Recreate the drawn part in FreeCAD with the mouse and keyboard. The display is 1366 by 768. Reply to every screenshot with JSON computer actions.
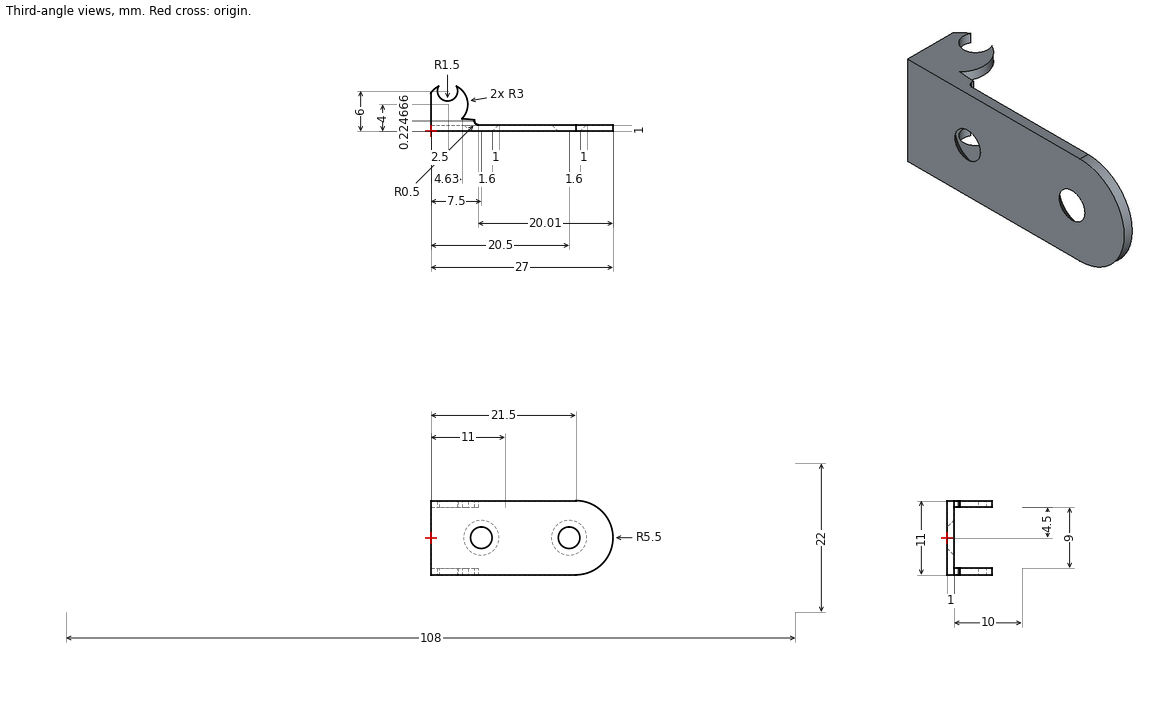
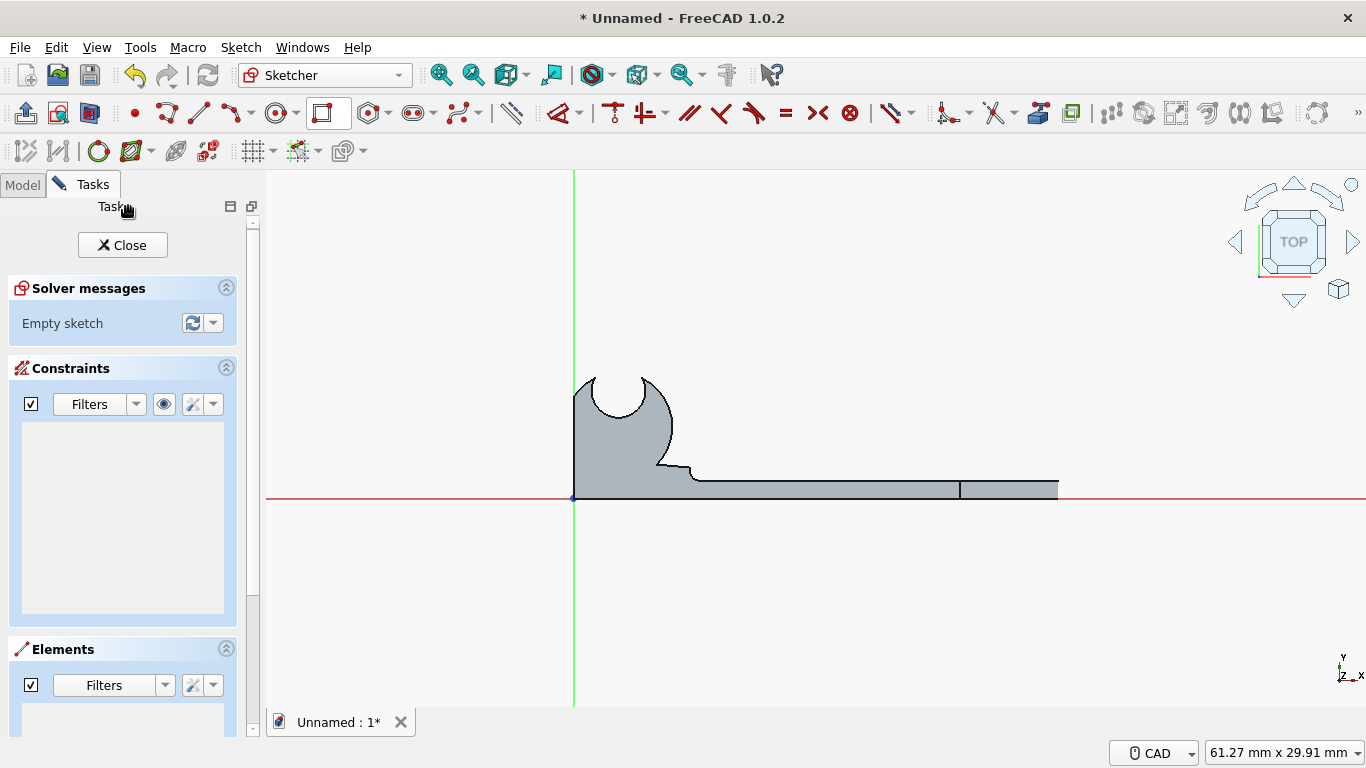
{"action": "key", "text": "q s"}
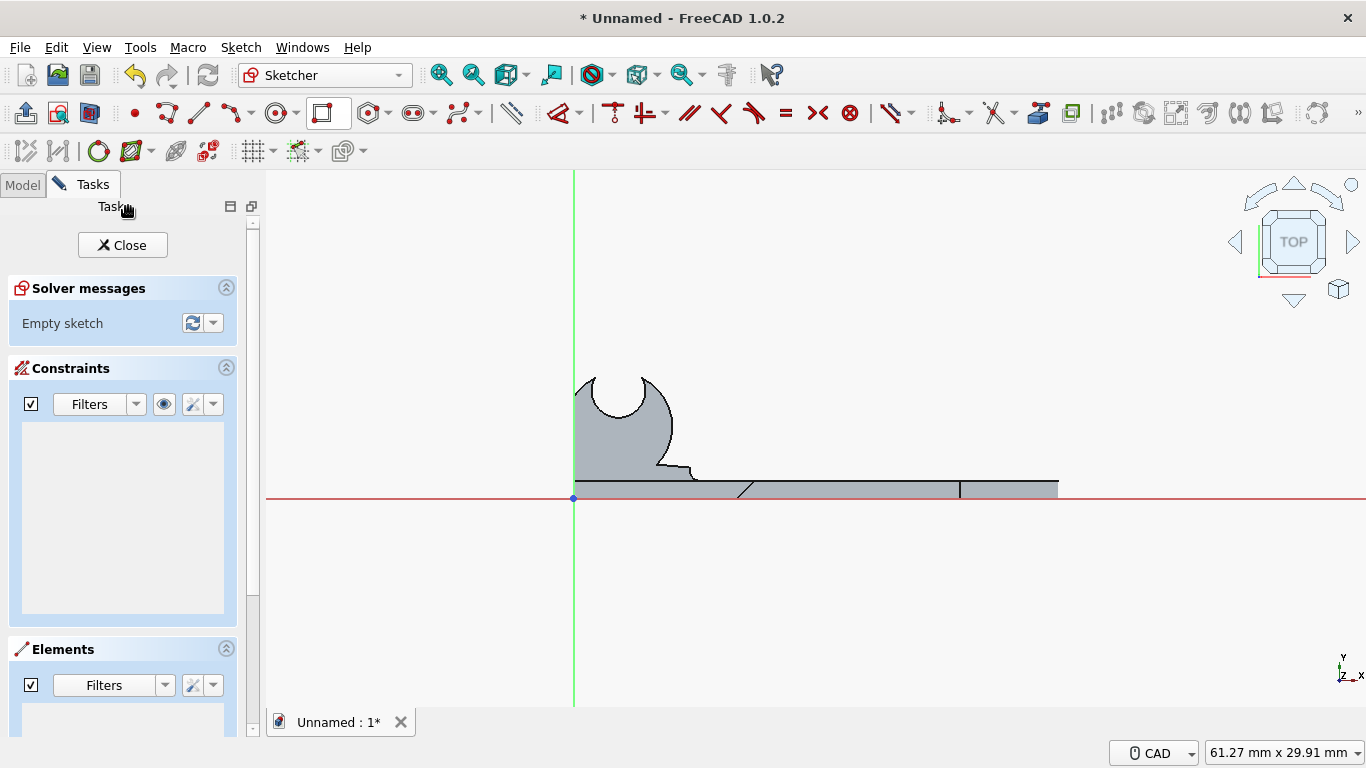
{"action": "scroll", "coordinate": [982, 490], "scroll_direction": "up", "scroll_amount": 13}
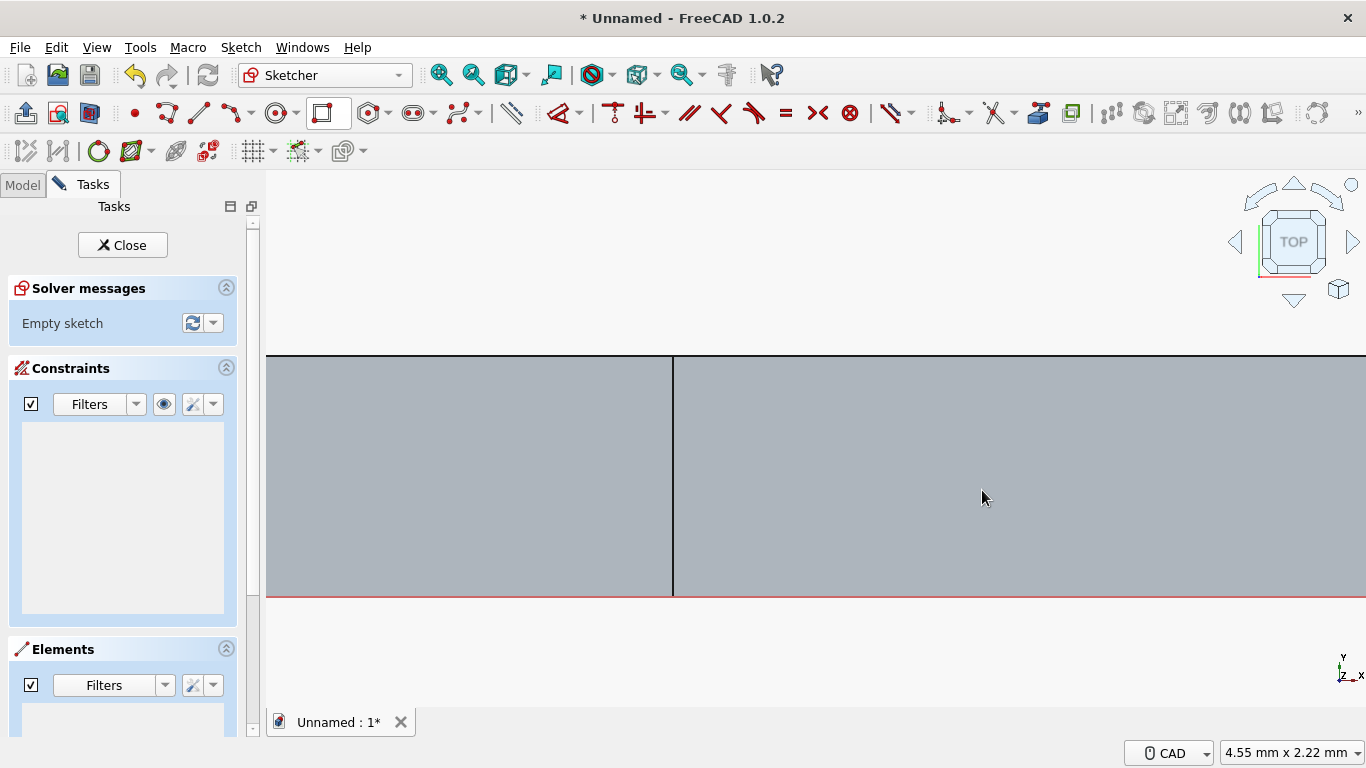
{"action": "key", "text": "g m"}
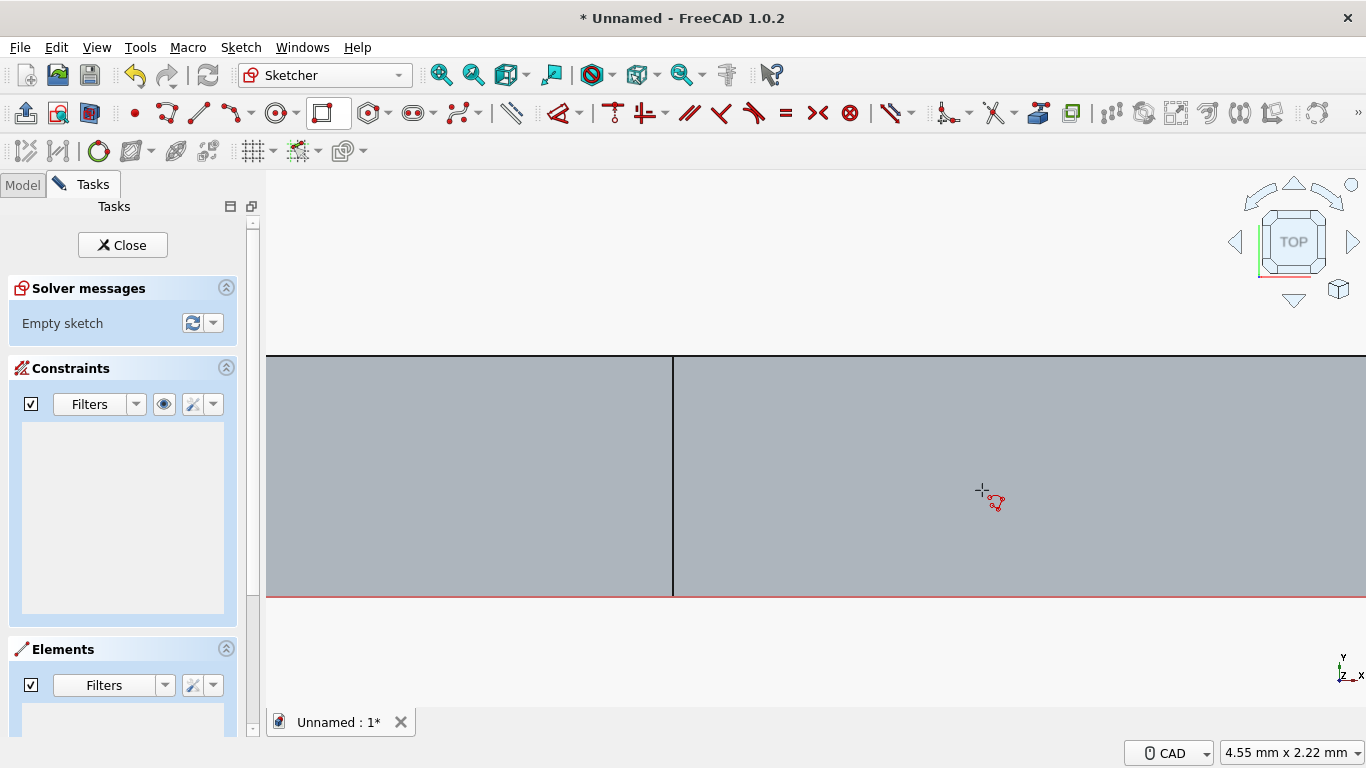
{"action": "left_click", "coordinate": [431, 597]}
{"action": "left_click", "coordinate": [818, 588]}
{"action": "left_click", "coordinate": [1059, 356]}
{"action": "left_click", "coordinate": [431, 356]}
{"action": "left_click", "coordinate": [431, 597]}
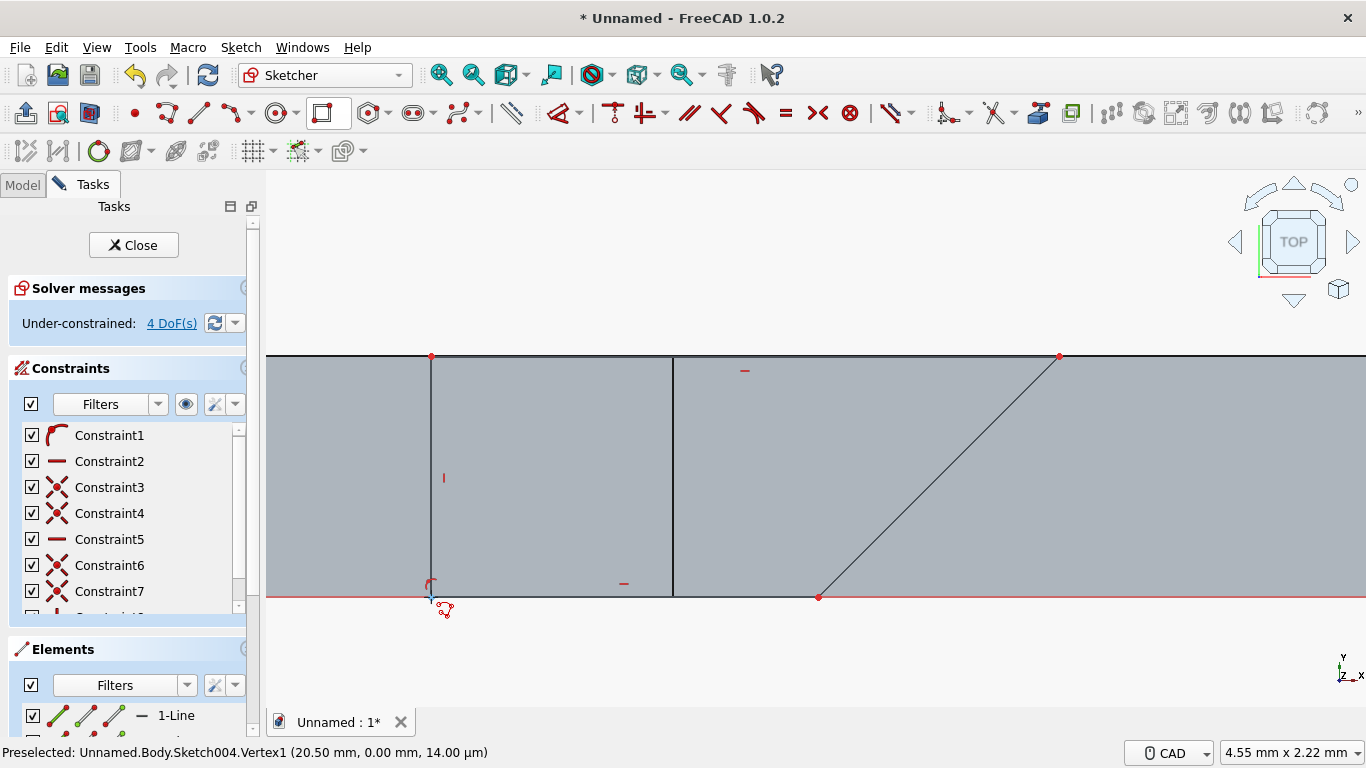
{"action": "key", "text": "g l"}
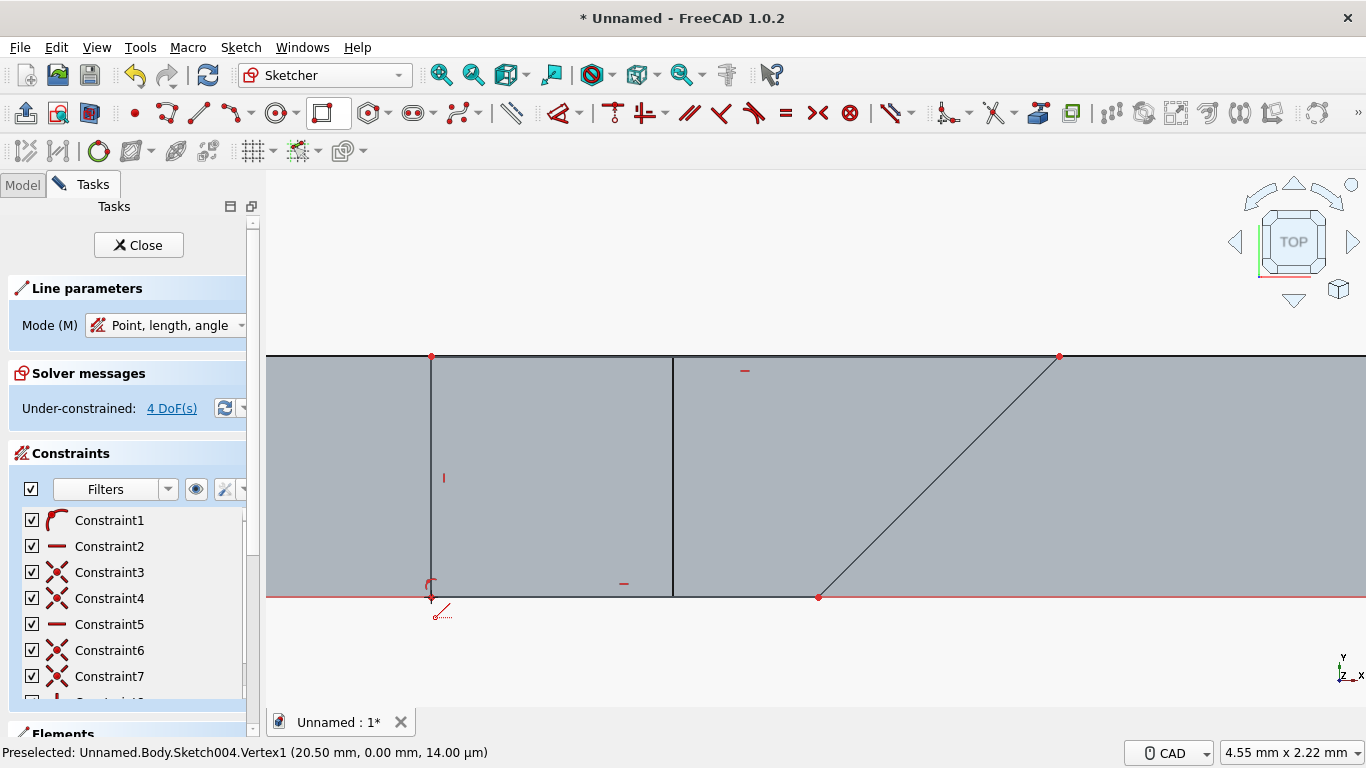
{"action": "left_click", "coordinate": [431, 331]}
{"action": "left_click", "coordinate": [431, 255]}
{"action": "key", "text": "Escape"}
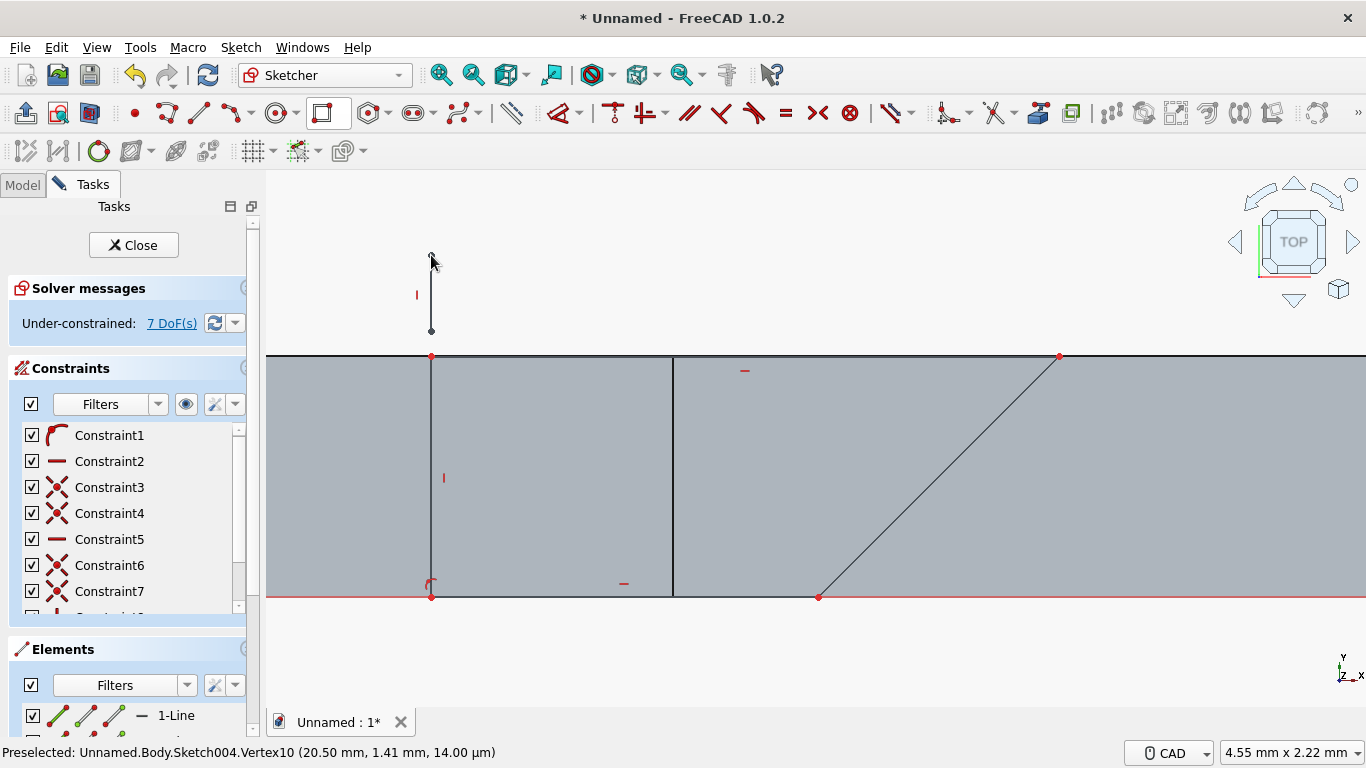
{"action": "left_click", "coordinate": [431, 309]}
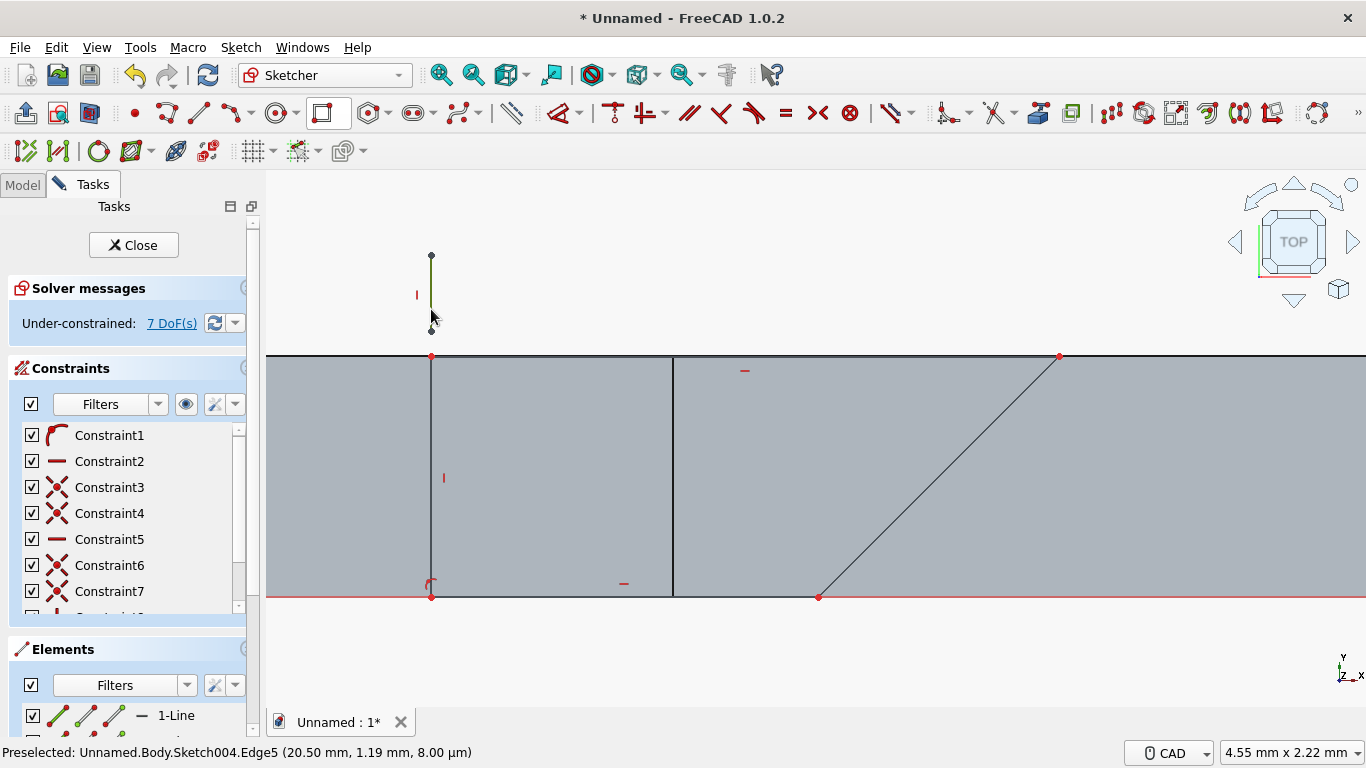
{"action": "key", "text": "g n"}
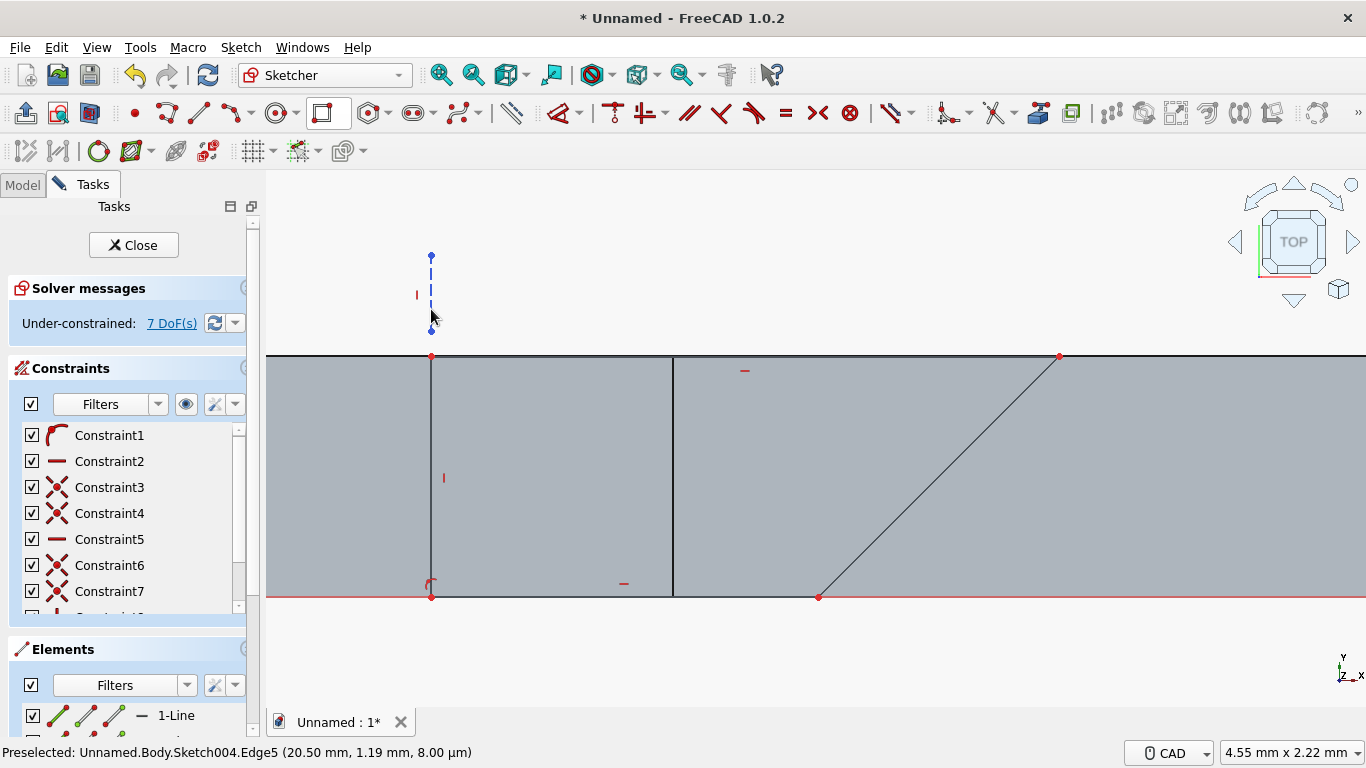
{"action": "key", "text": "d"}